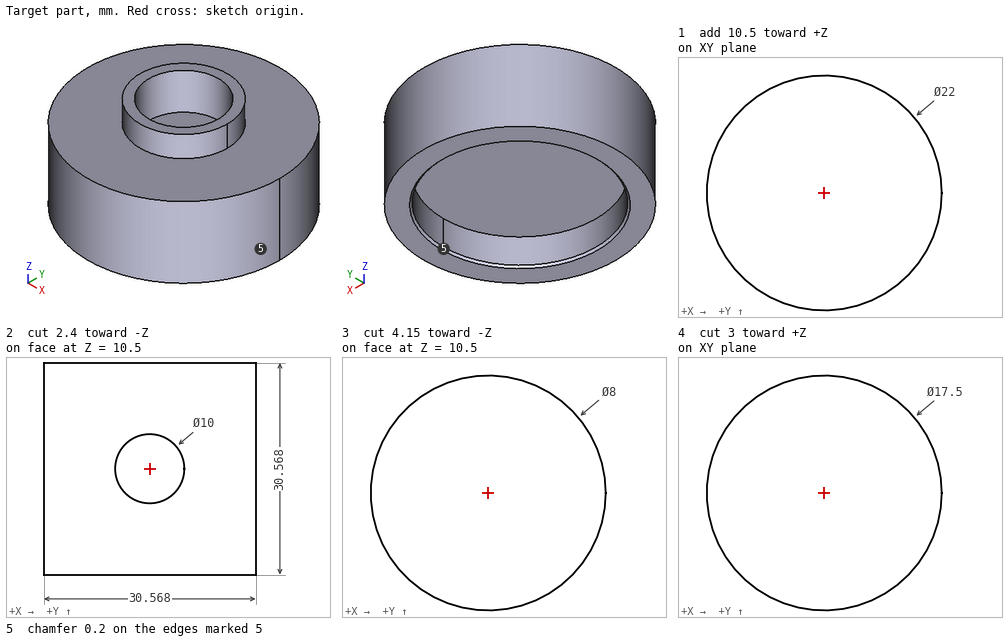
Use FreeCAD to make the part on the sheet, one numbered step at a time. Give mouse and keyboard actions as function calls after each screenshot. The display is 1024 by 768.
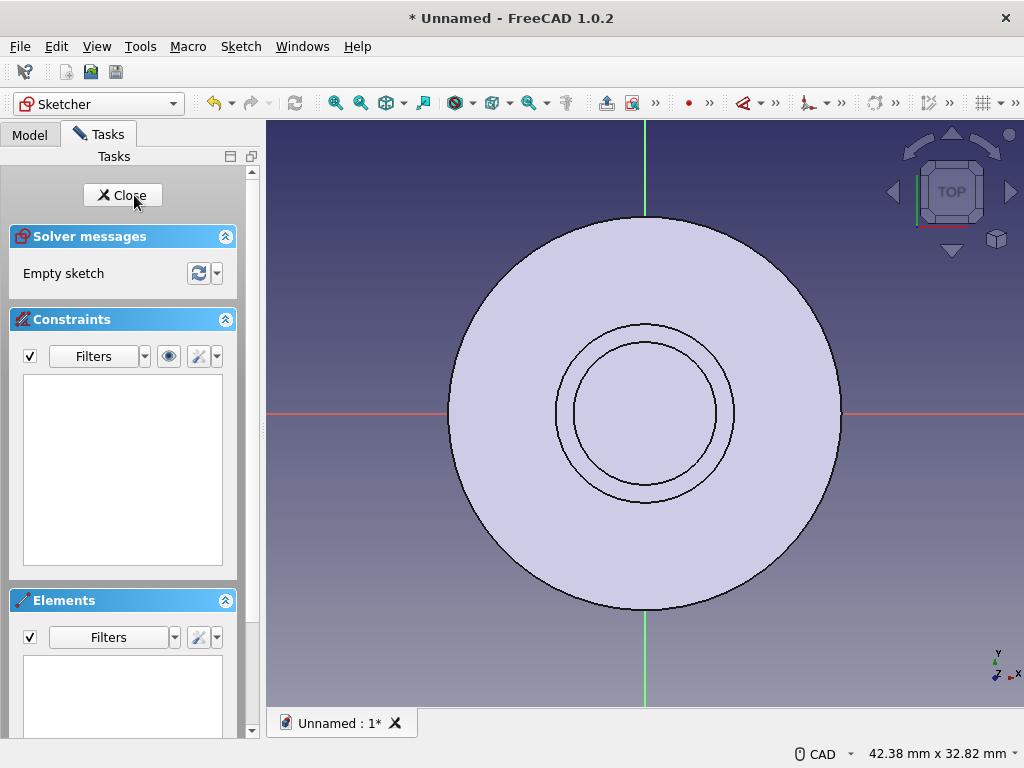
key(q)
key(s)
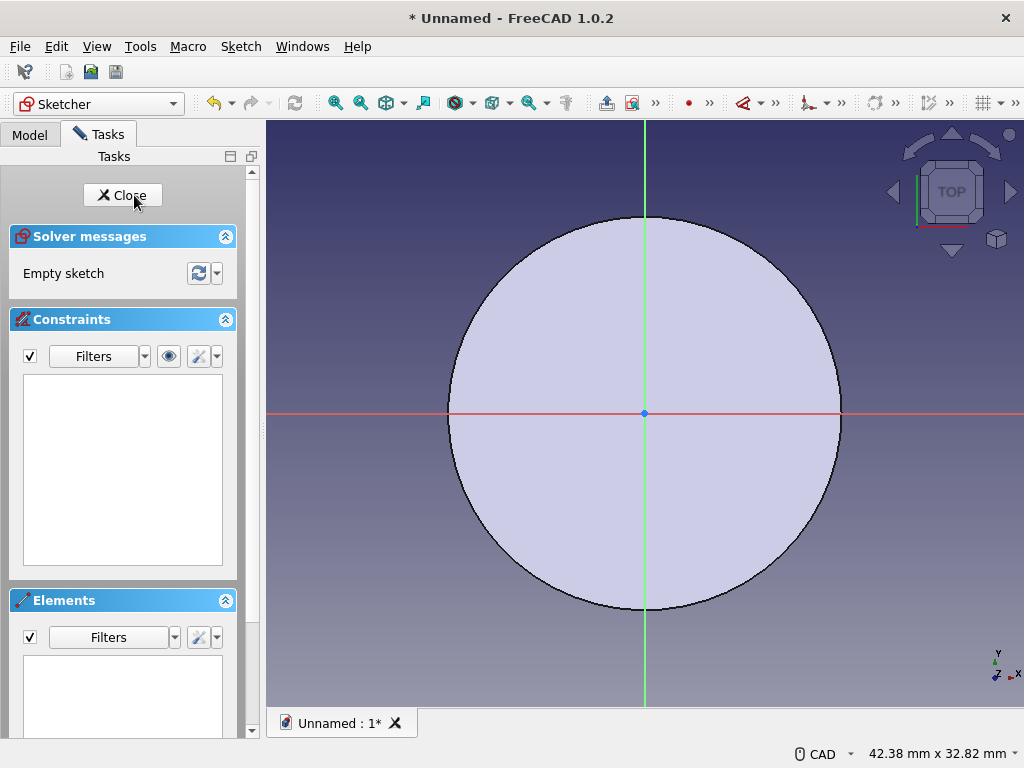
key(g)
key(c)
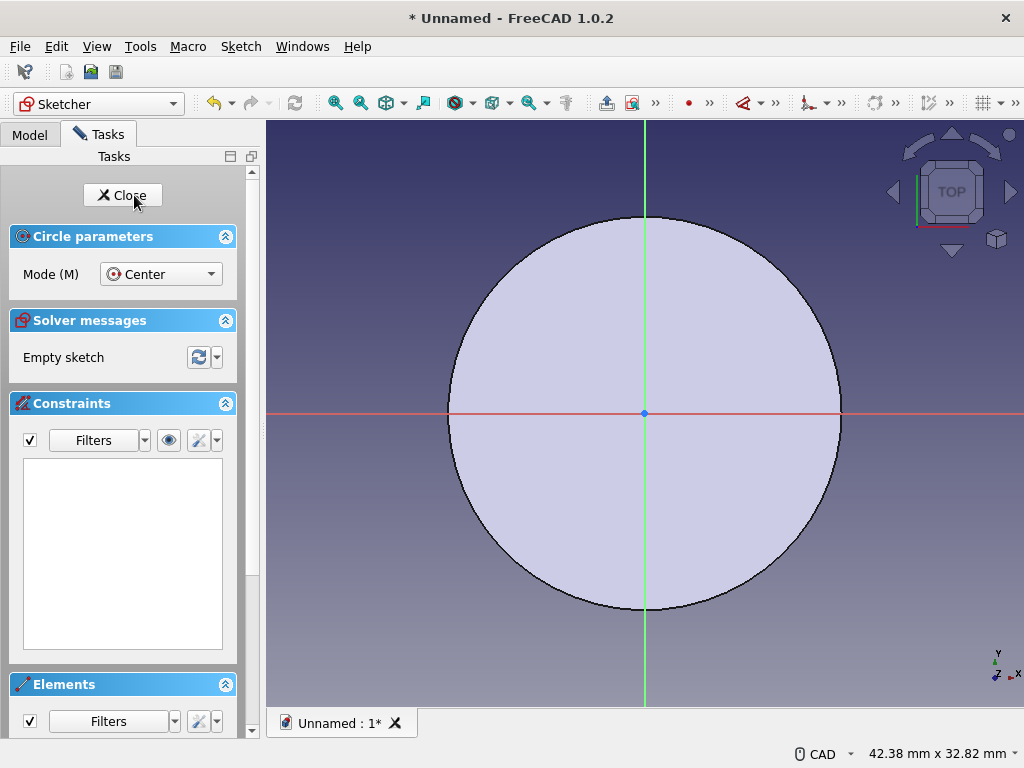
click(645, 414)
move(756, 303)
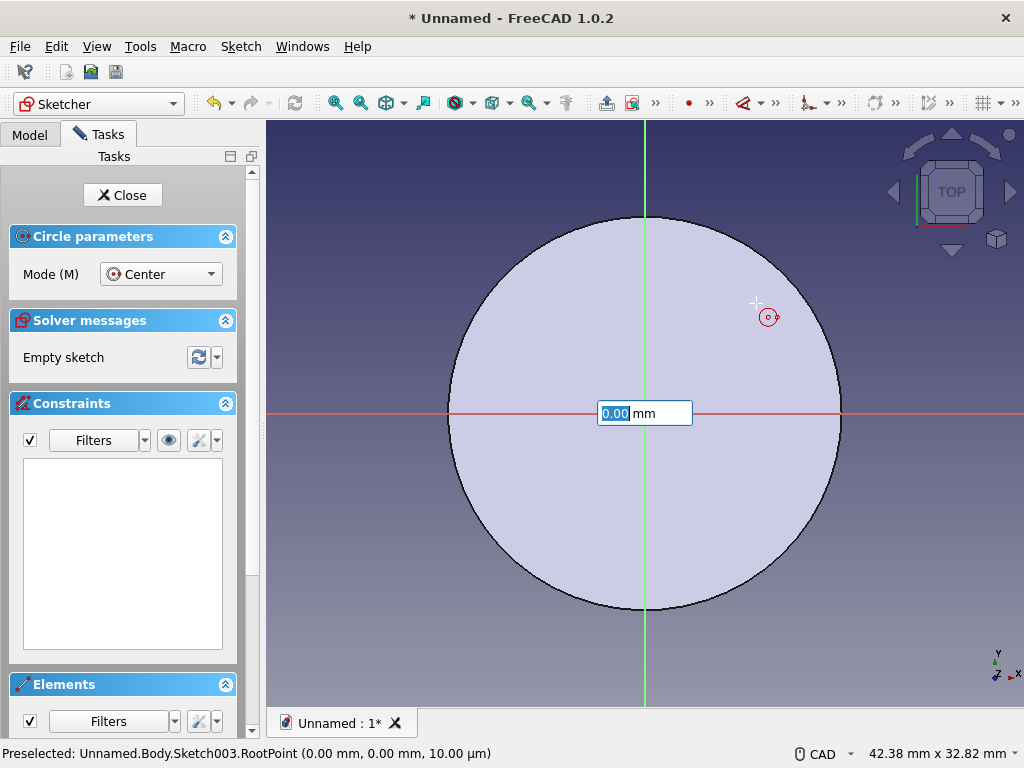
text(17.5)
key(Return)
key(Escape)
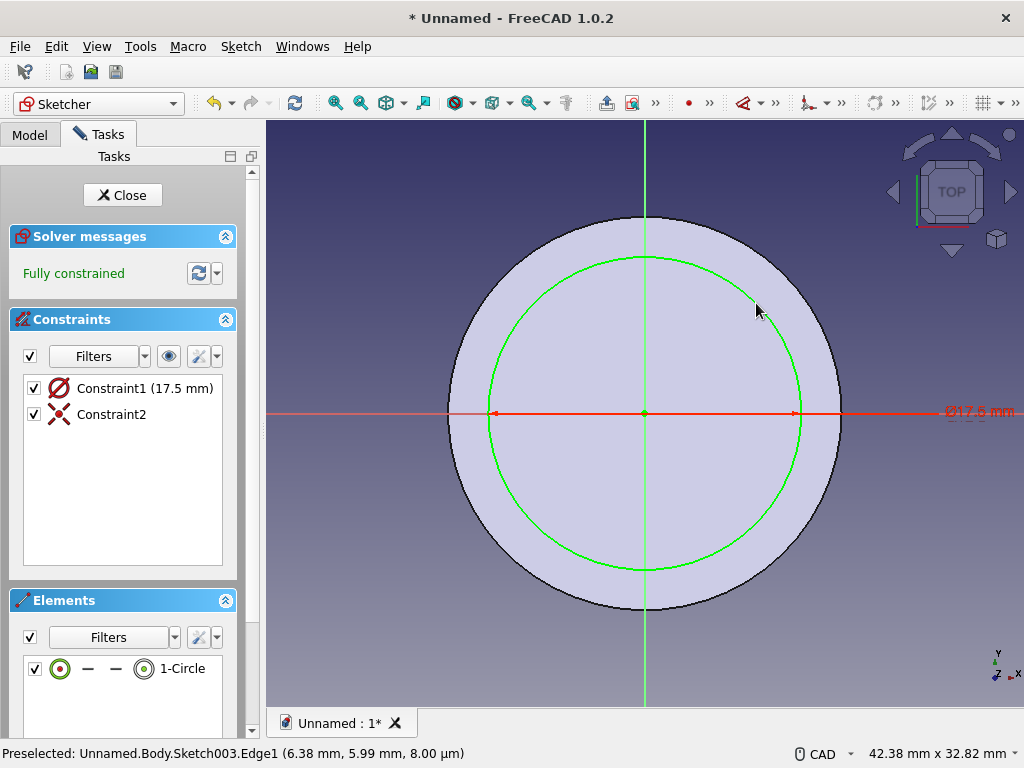
click(123, 195)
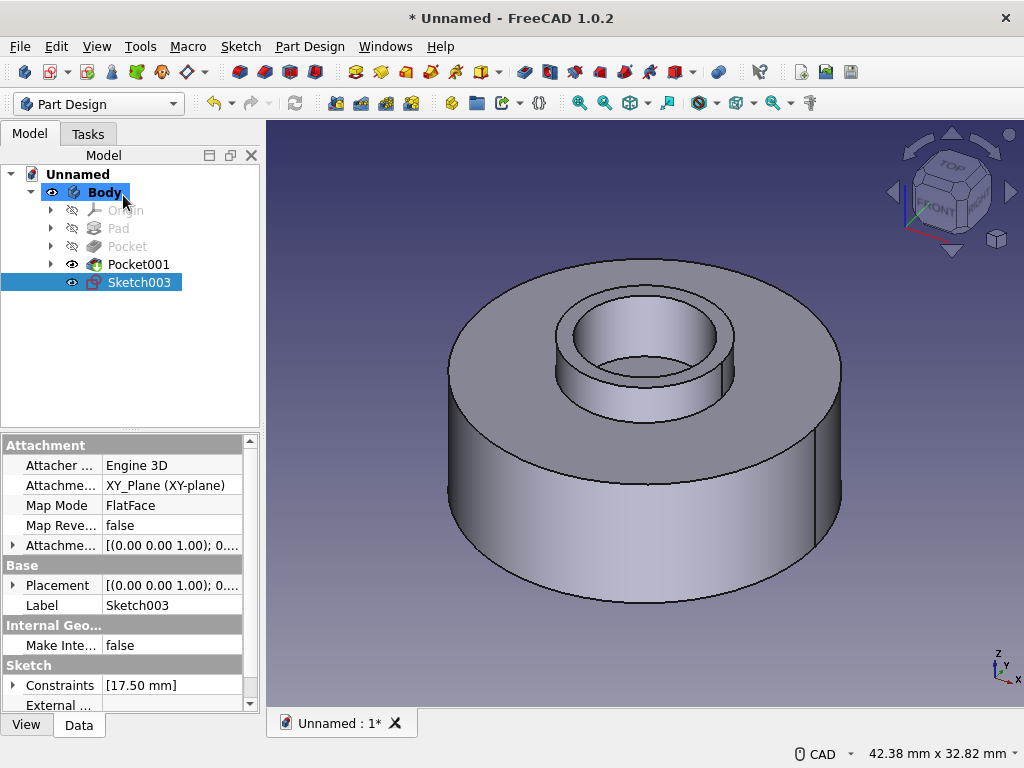
click(525, 72)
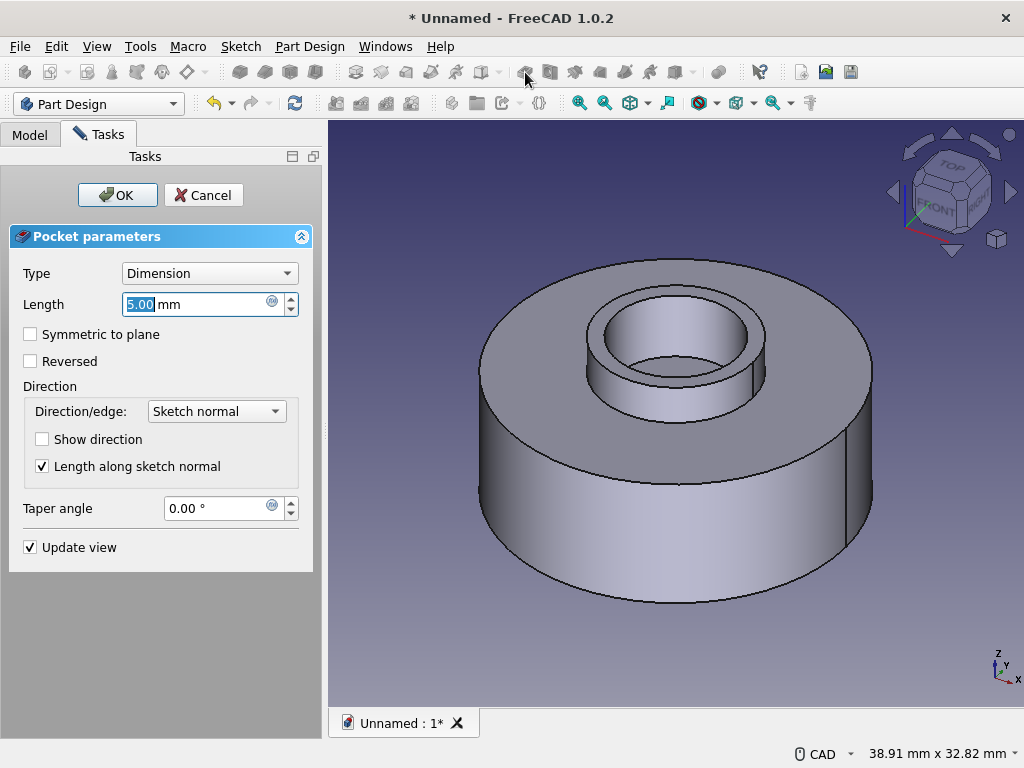
text(3)
key(Tab)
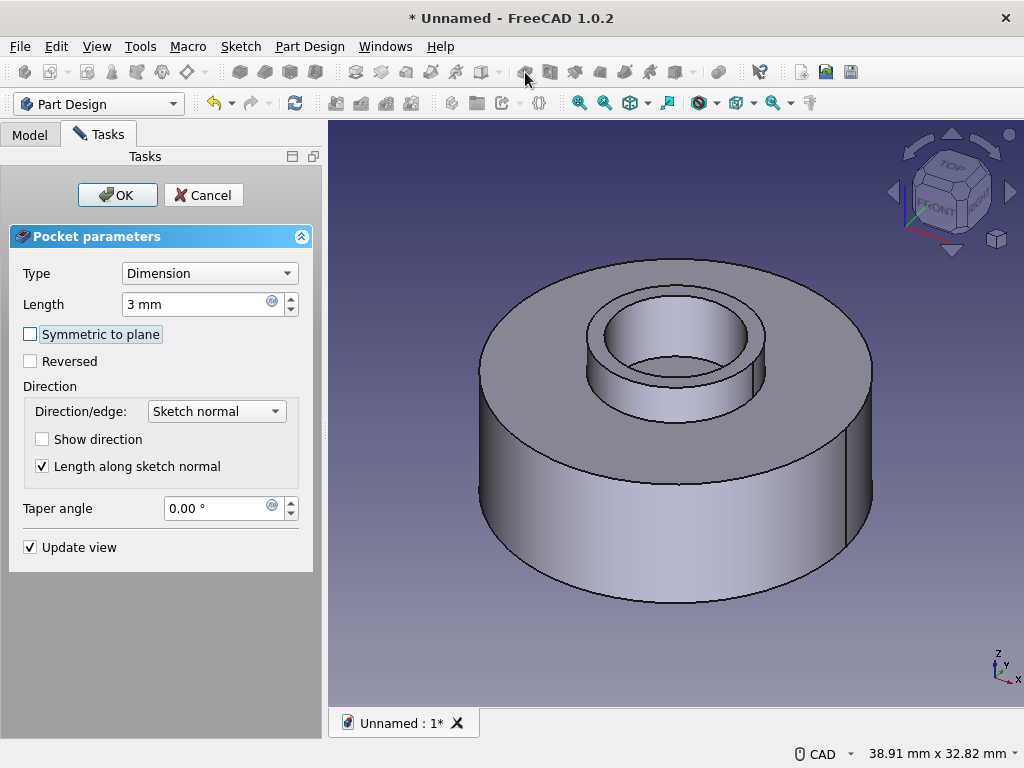
click(31, 361)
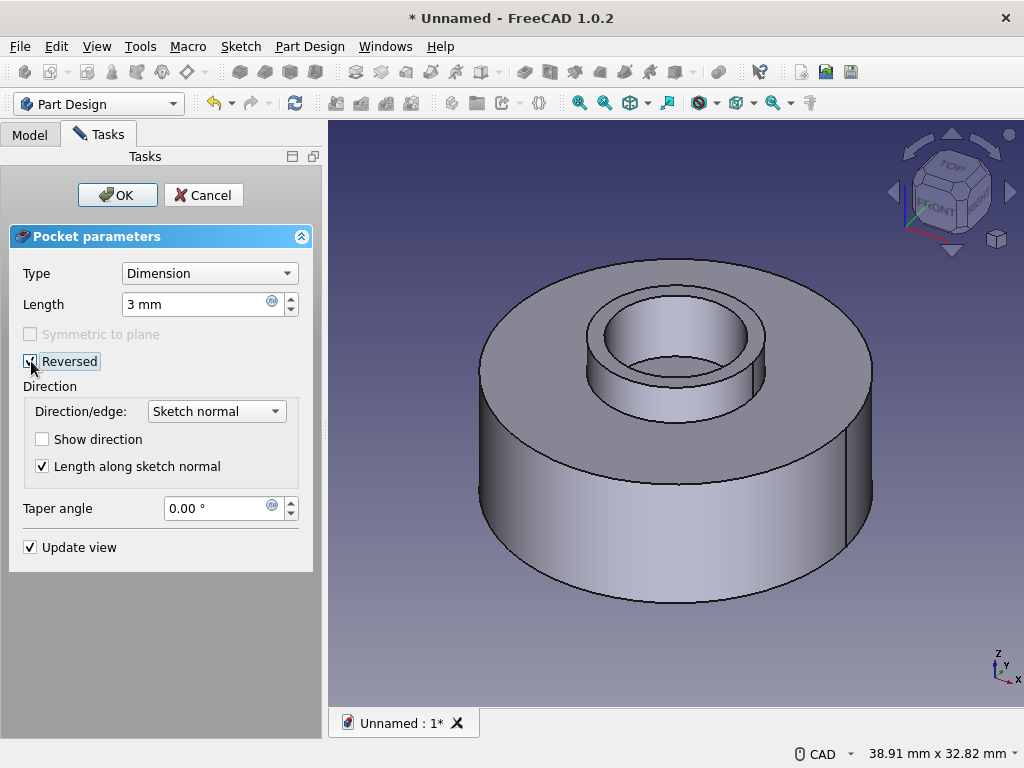
click(118, 195)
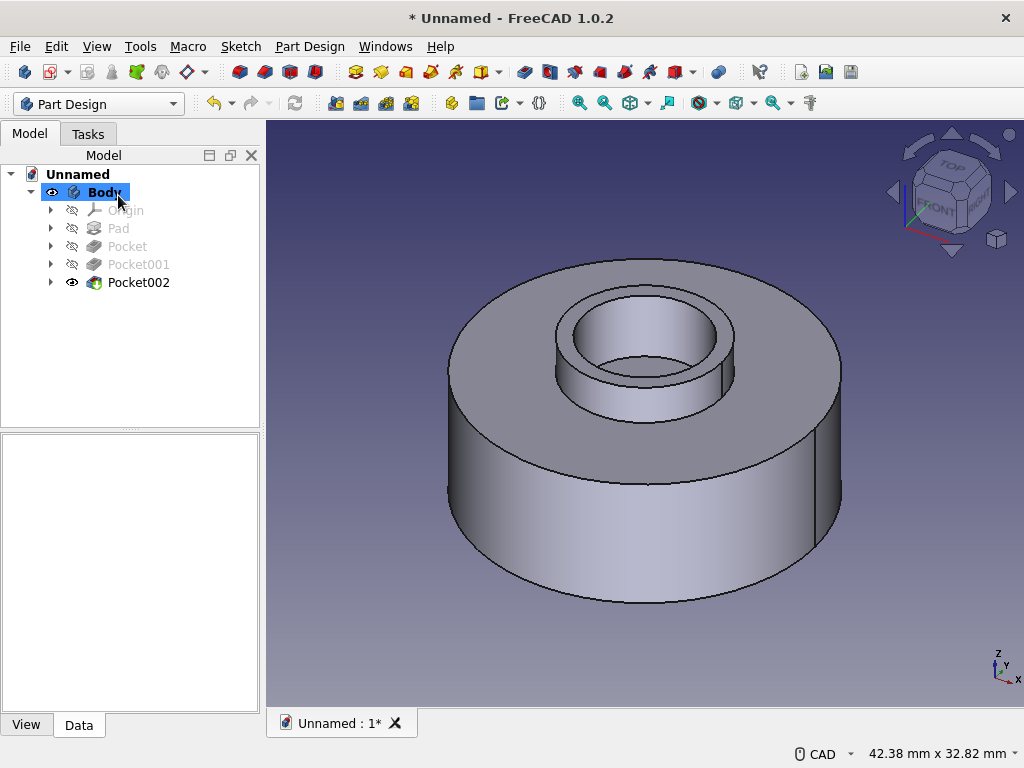
key(0)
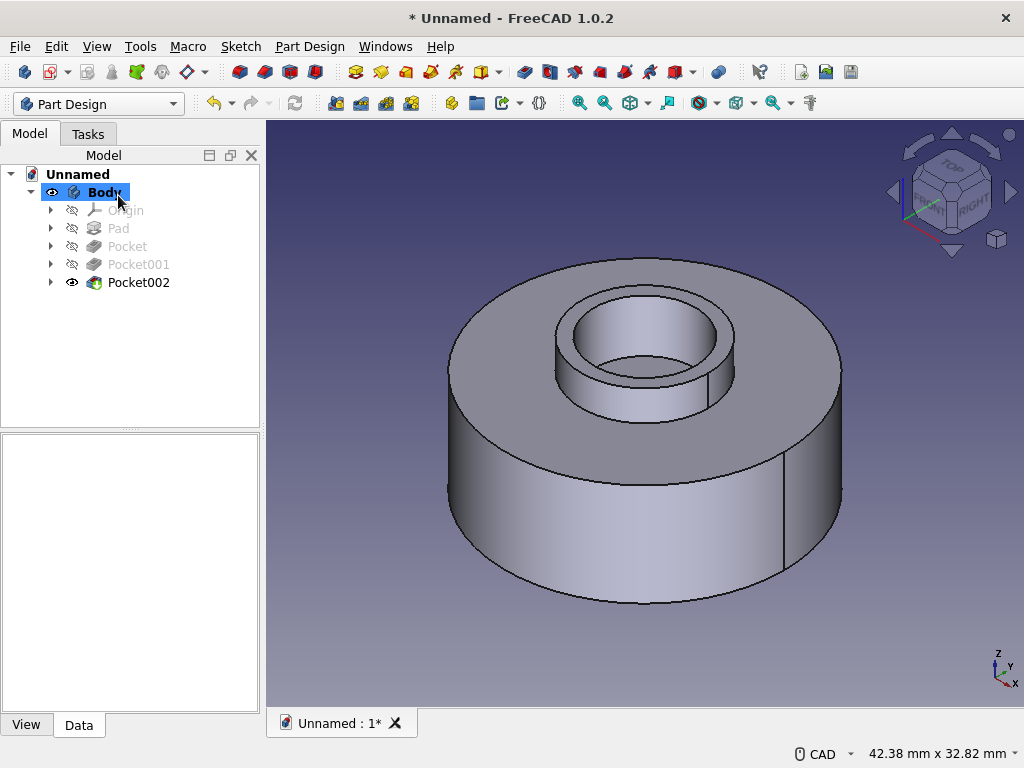
key(2)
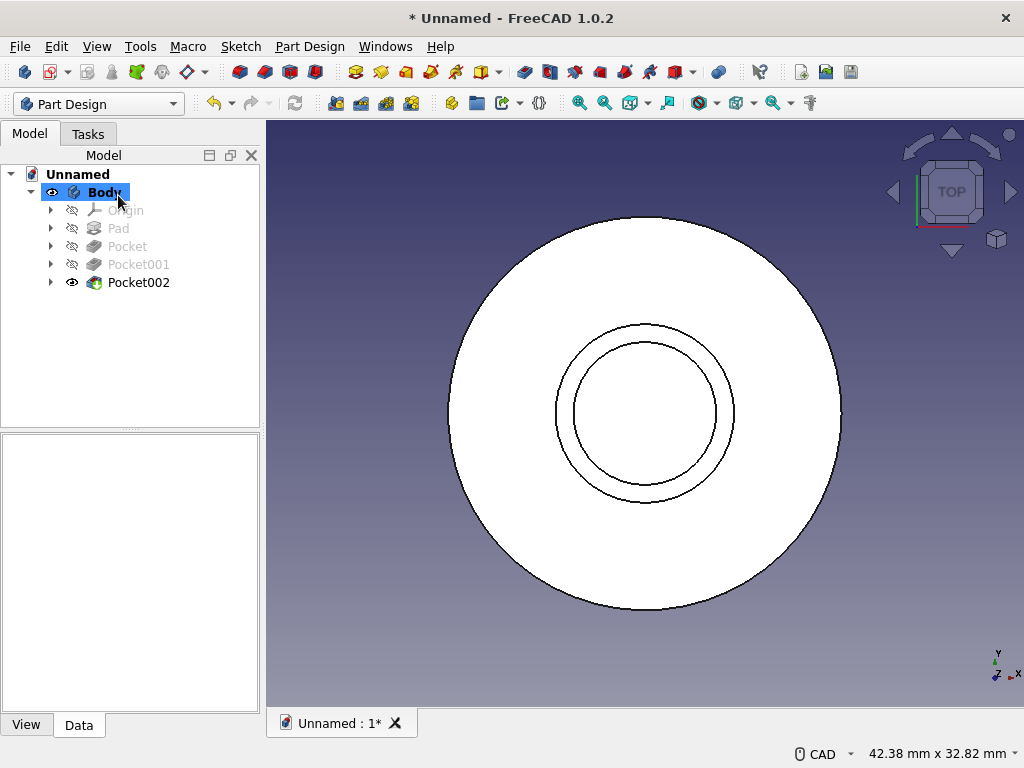
key(1)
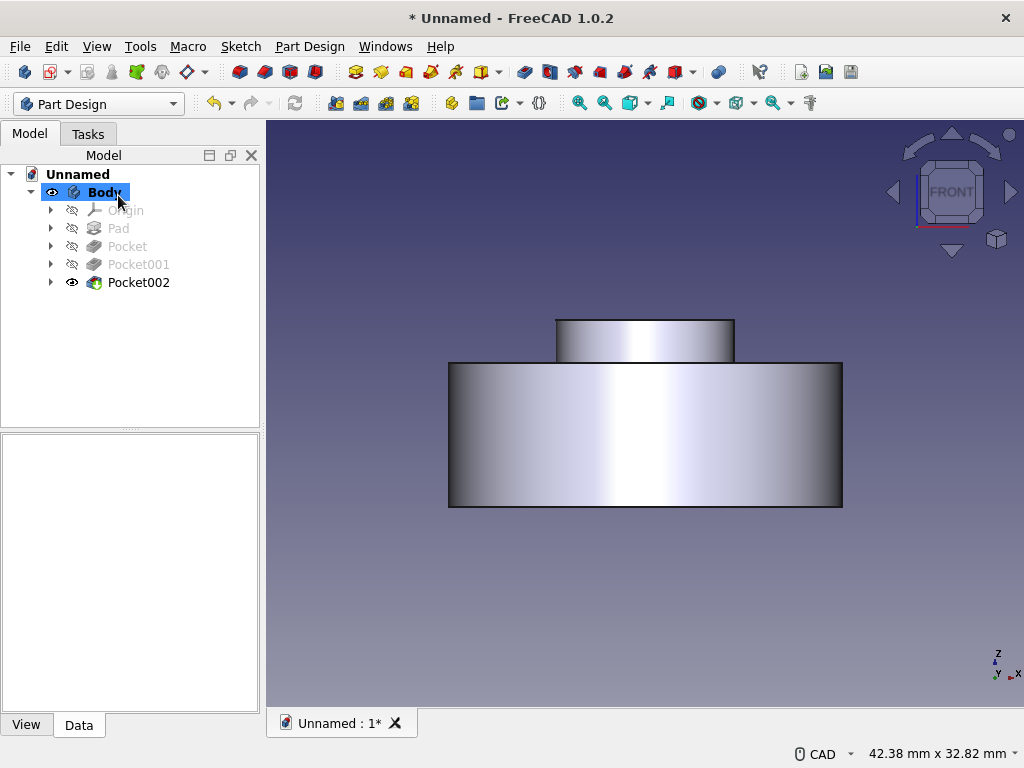
key(3)